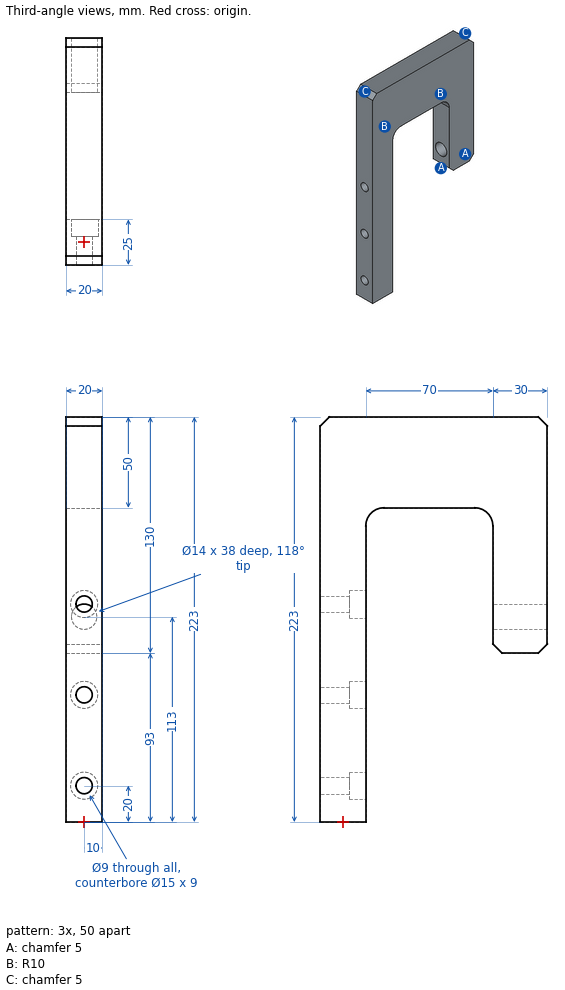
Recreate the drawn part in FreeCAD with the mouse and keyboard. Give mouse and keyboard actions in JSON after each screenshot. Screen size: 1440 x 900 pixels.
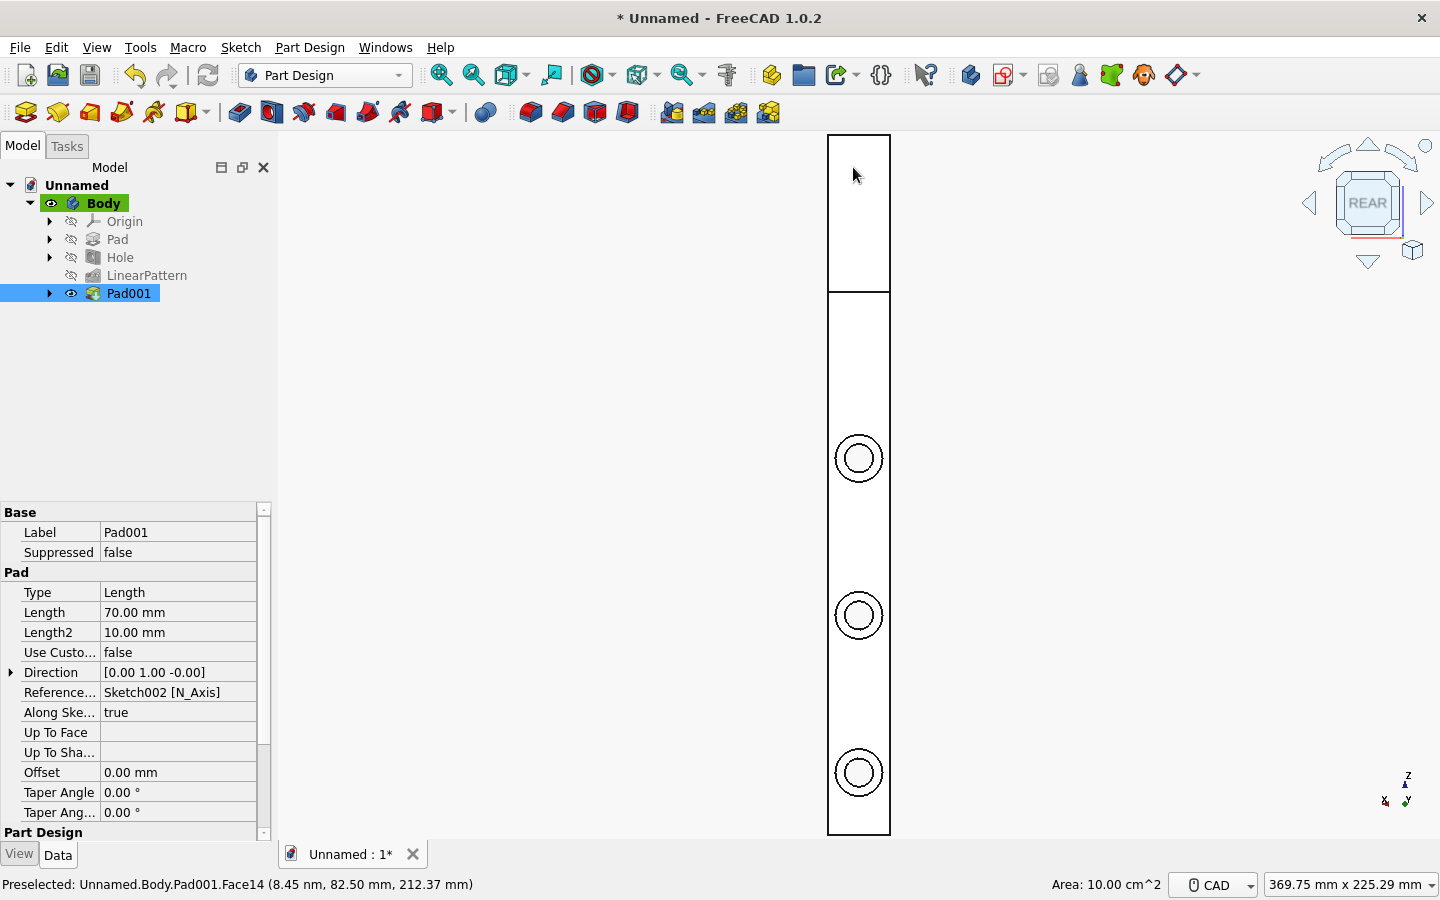
{"action": "left_click", "coordinate": [1004, 76]}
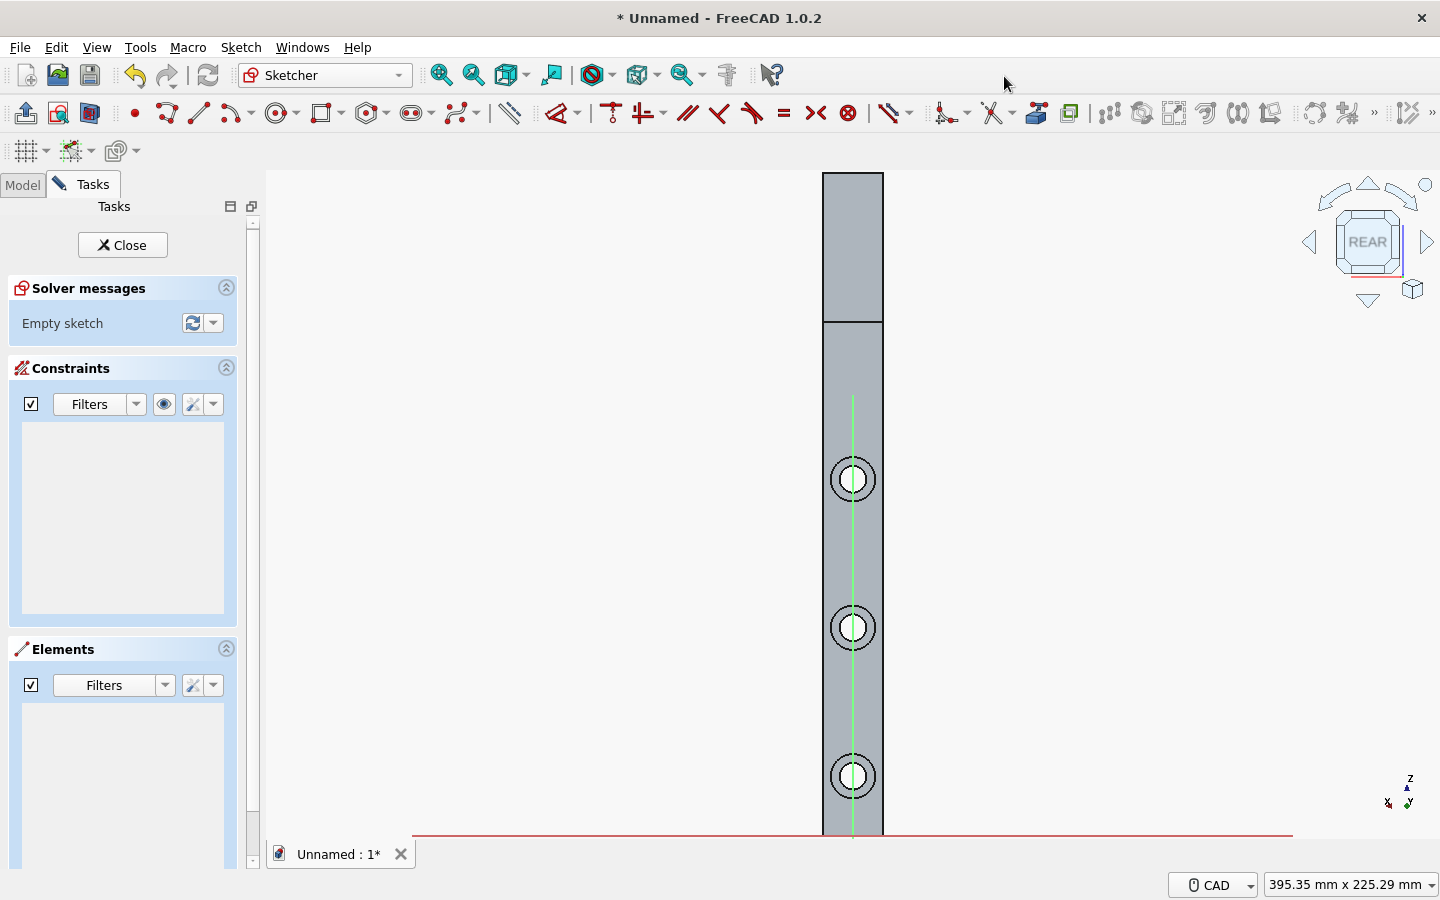
{"action": "scroll", "coordinate": [645, 504], "scroll_direction": "down", "scroll_amount": 2}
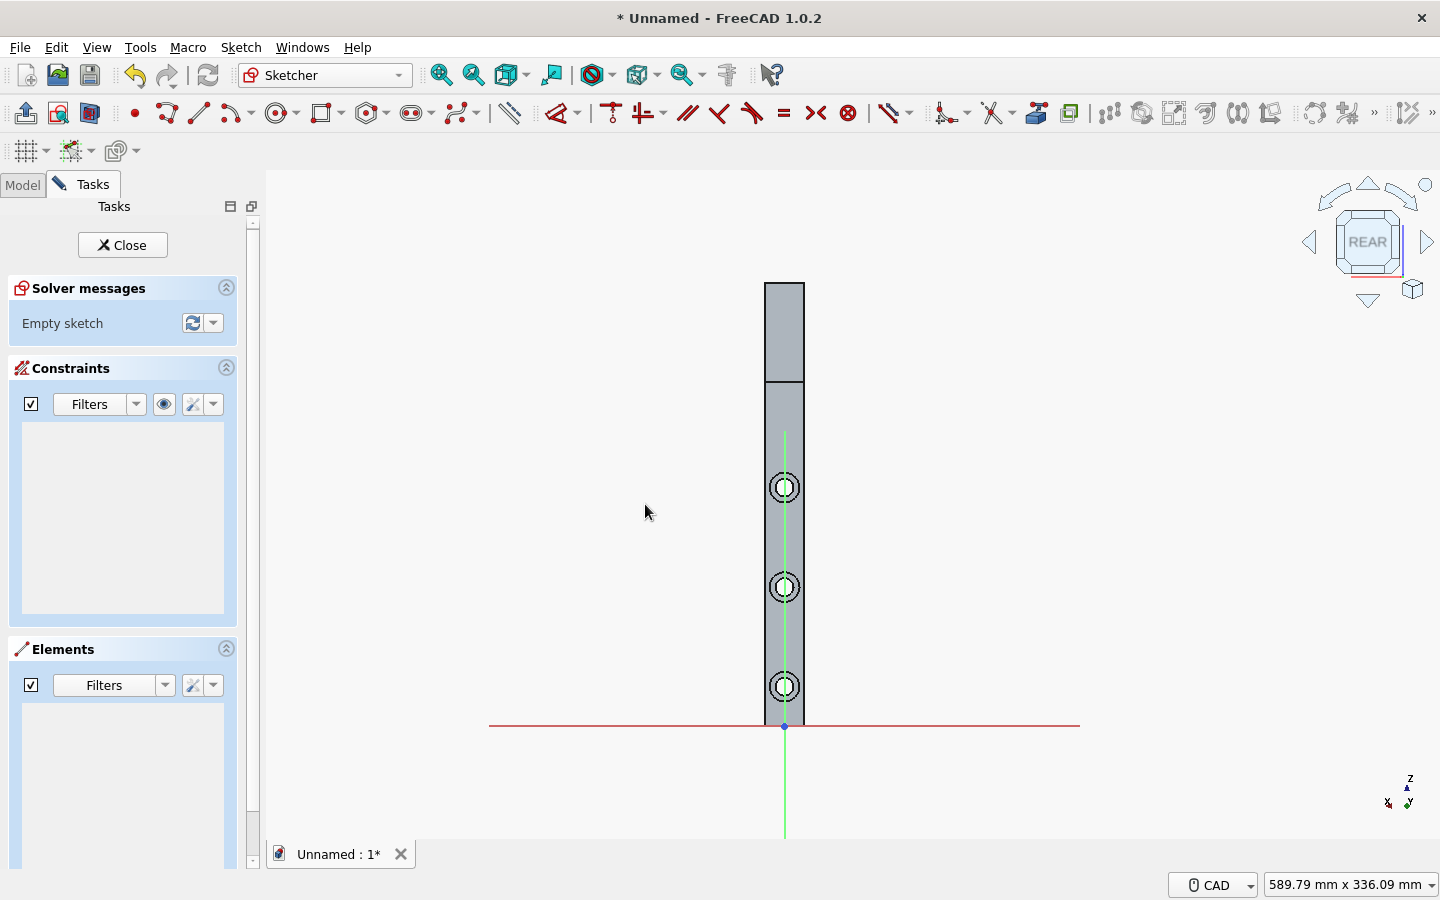
{"action": "left_click", "coordinate": [322, 114]}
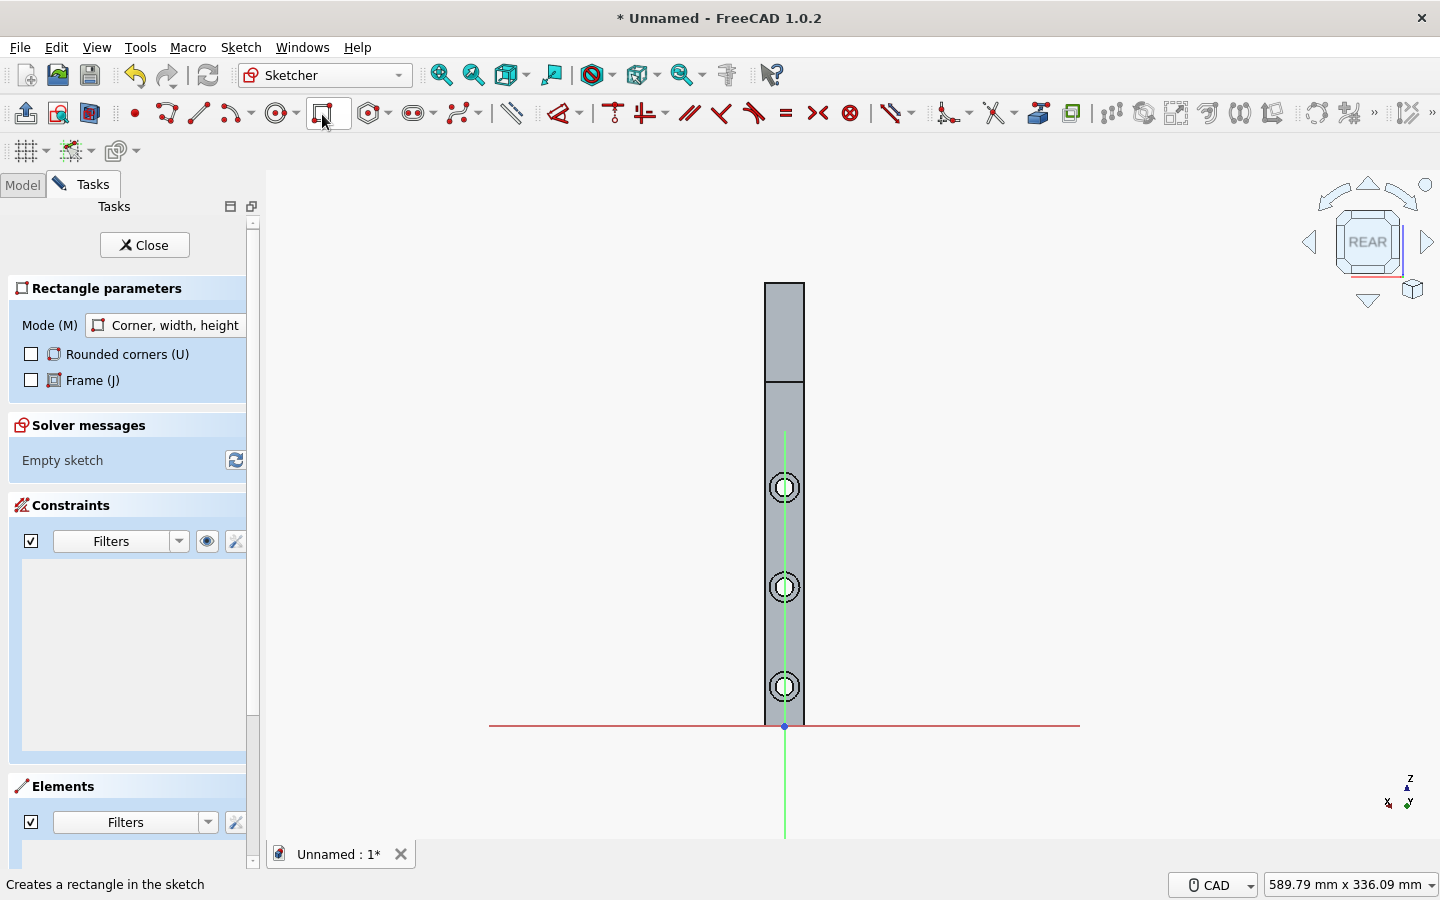
{"action": "left_click", "coordinate": [765, 283]}
{"action": "left_click", "coordinate": [804, 541]}
{"action": "key", "text": "Escape"}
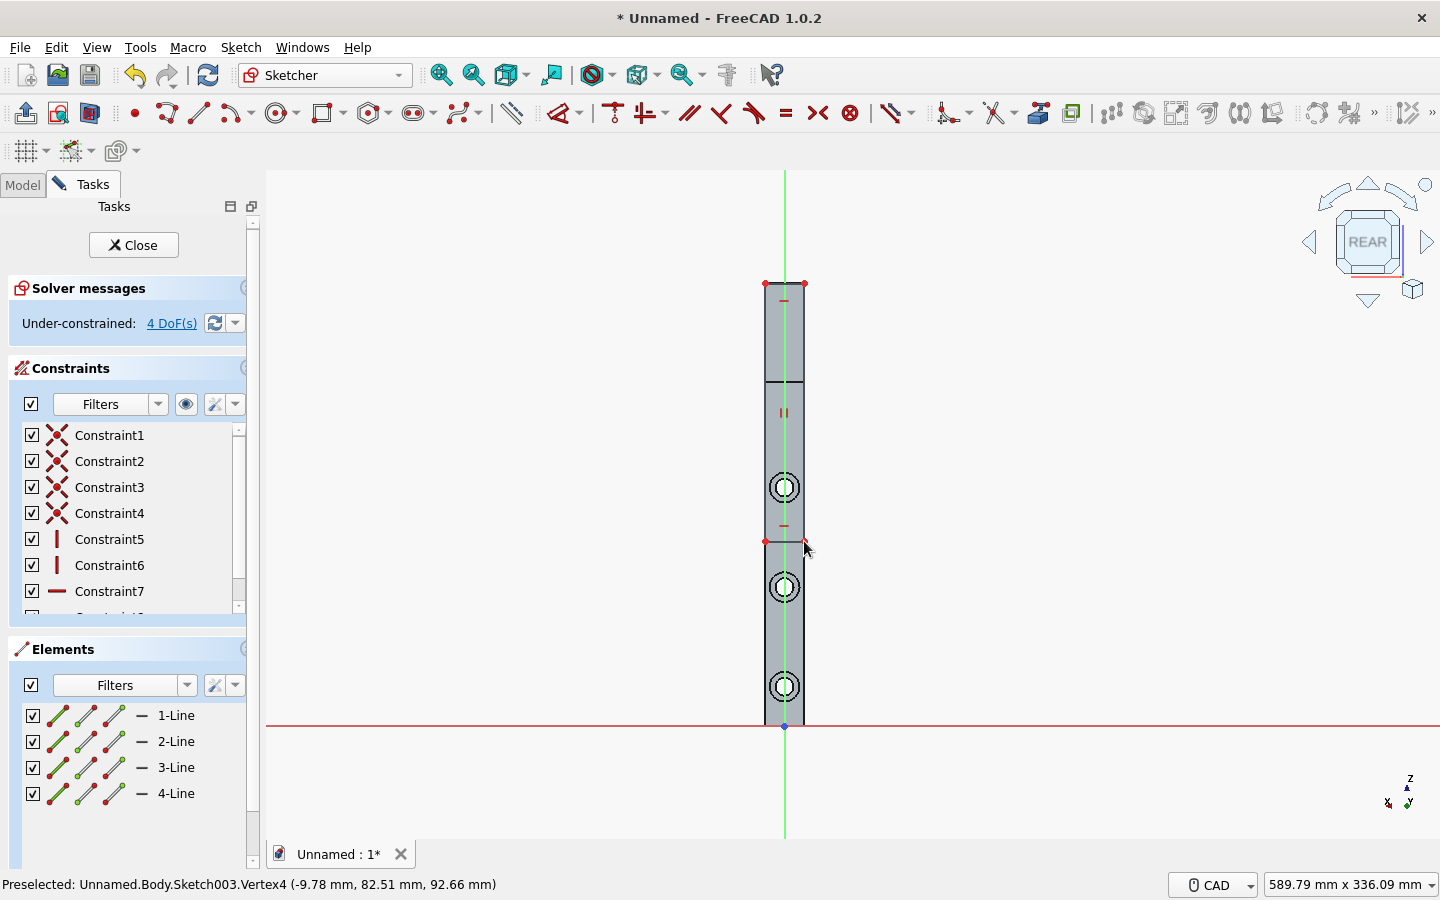
{"action": "left_click", "coordinate": [558, 114]}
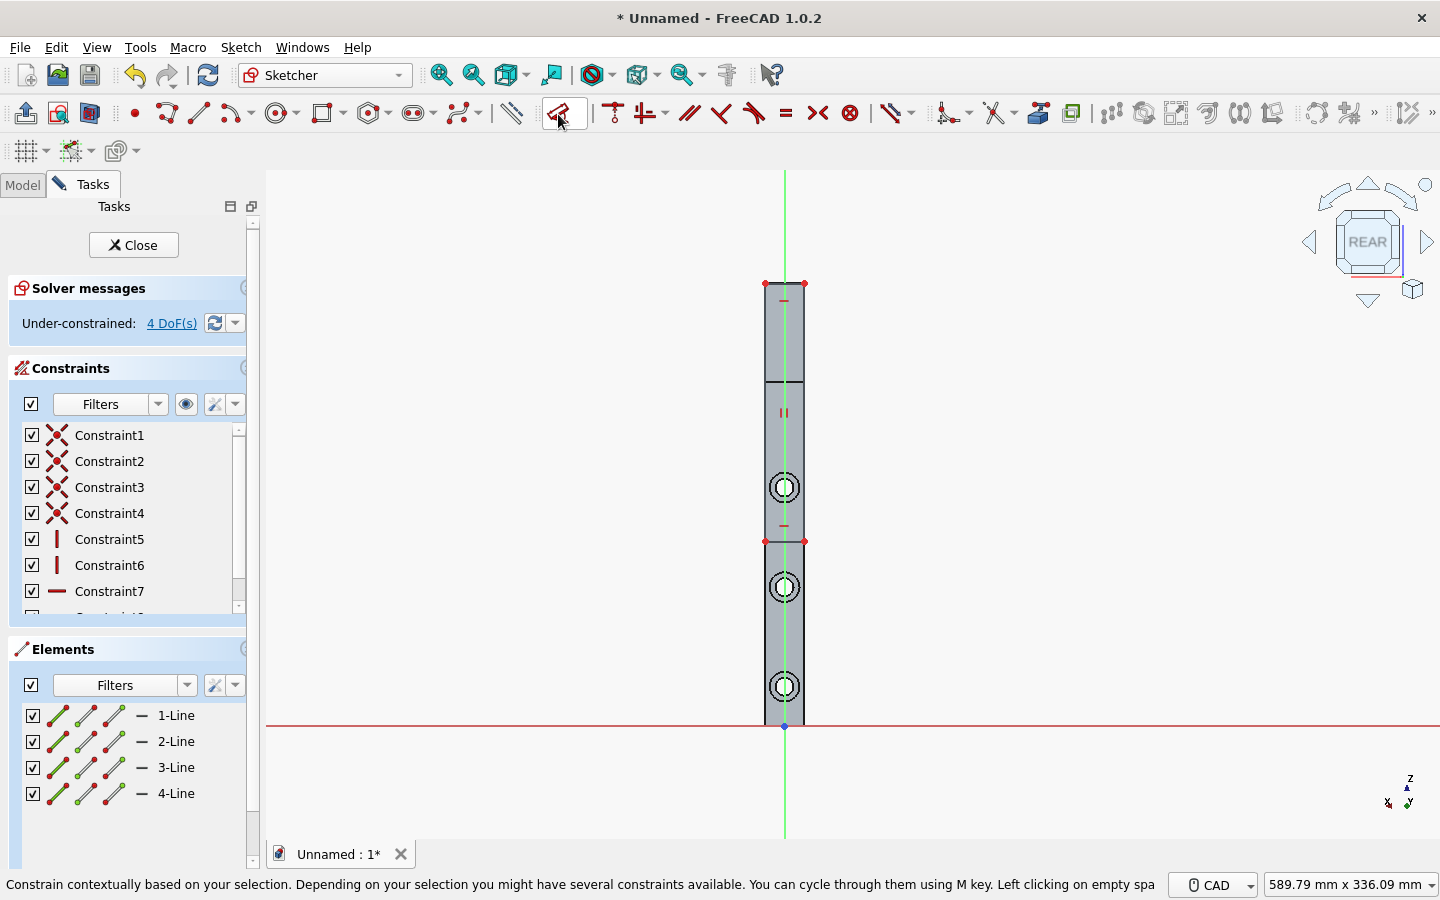
{"action": "left_click", "coordinate": [781, 542]}
{"action": "left_click", "coordinate": [771, 576]}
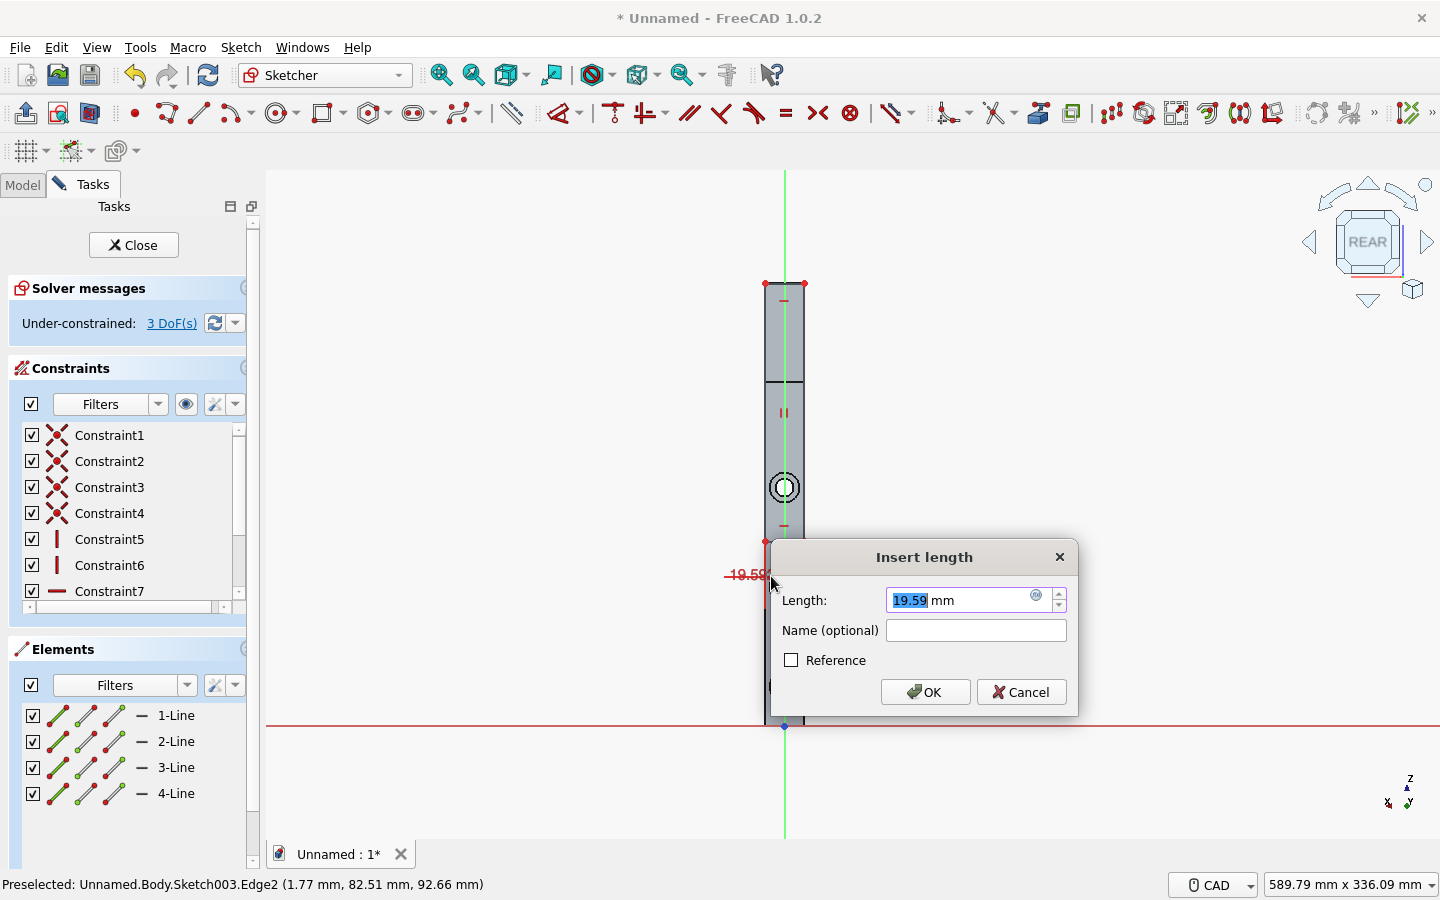
{"action": "type", "text": "20"}
{"action": "key", "text": "Return"}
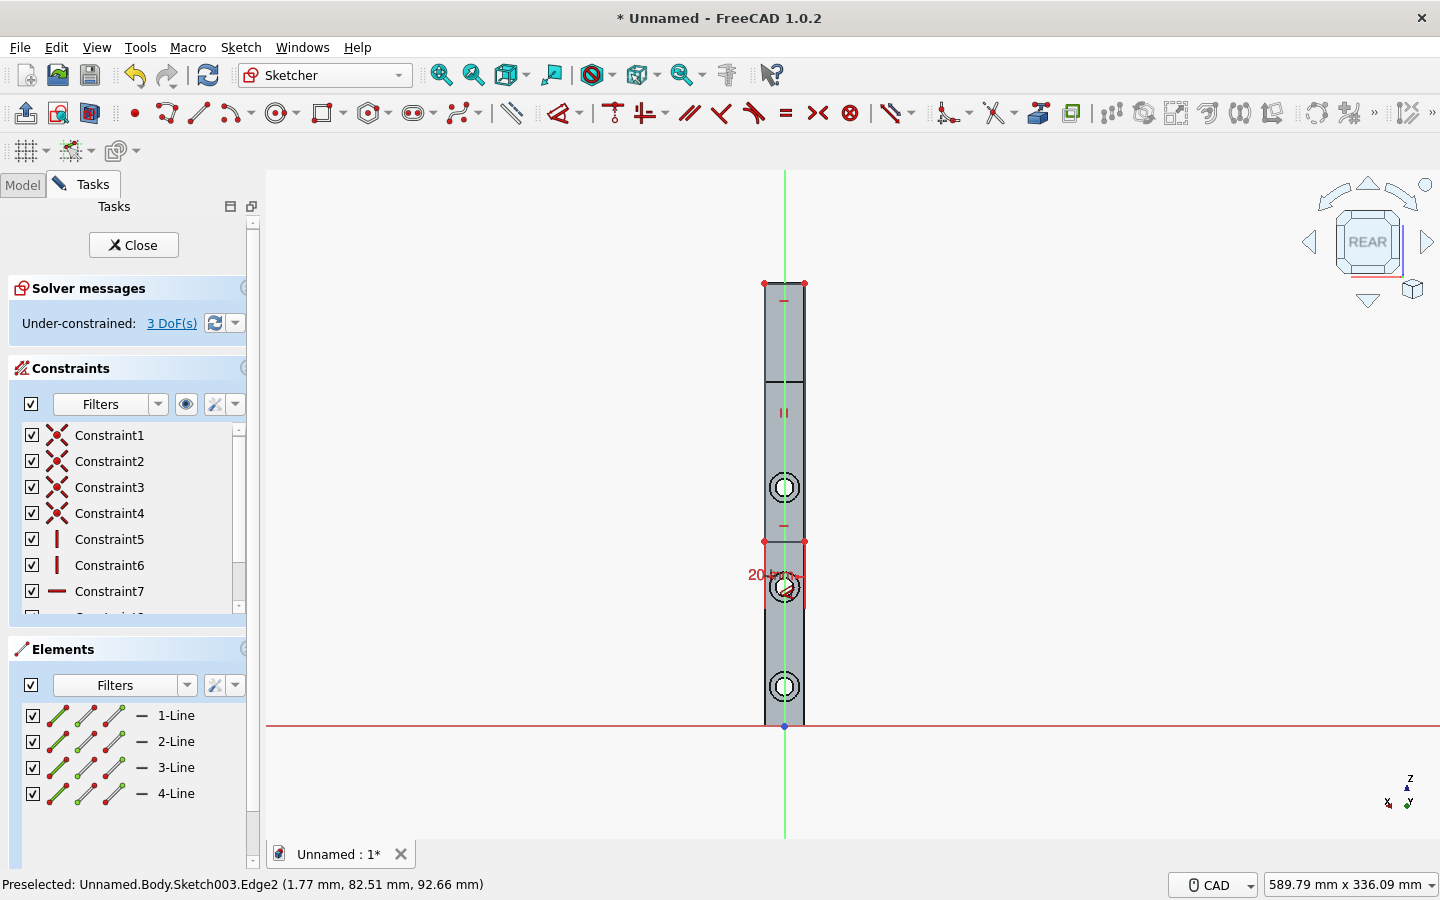
{"action": "left_click", "coordinate": [765, 361]}
{"action": "left_click", "coordinate": [731, 413]}